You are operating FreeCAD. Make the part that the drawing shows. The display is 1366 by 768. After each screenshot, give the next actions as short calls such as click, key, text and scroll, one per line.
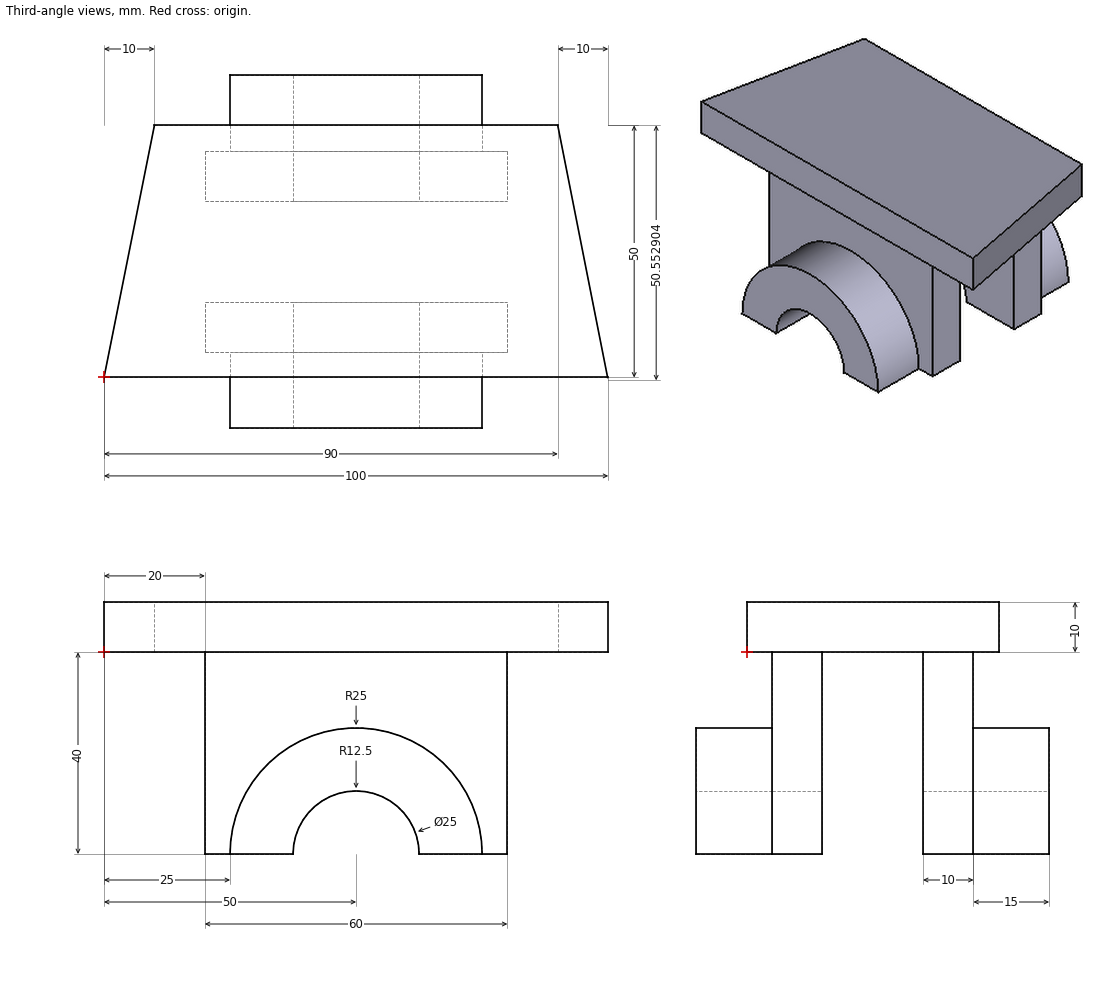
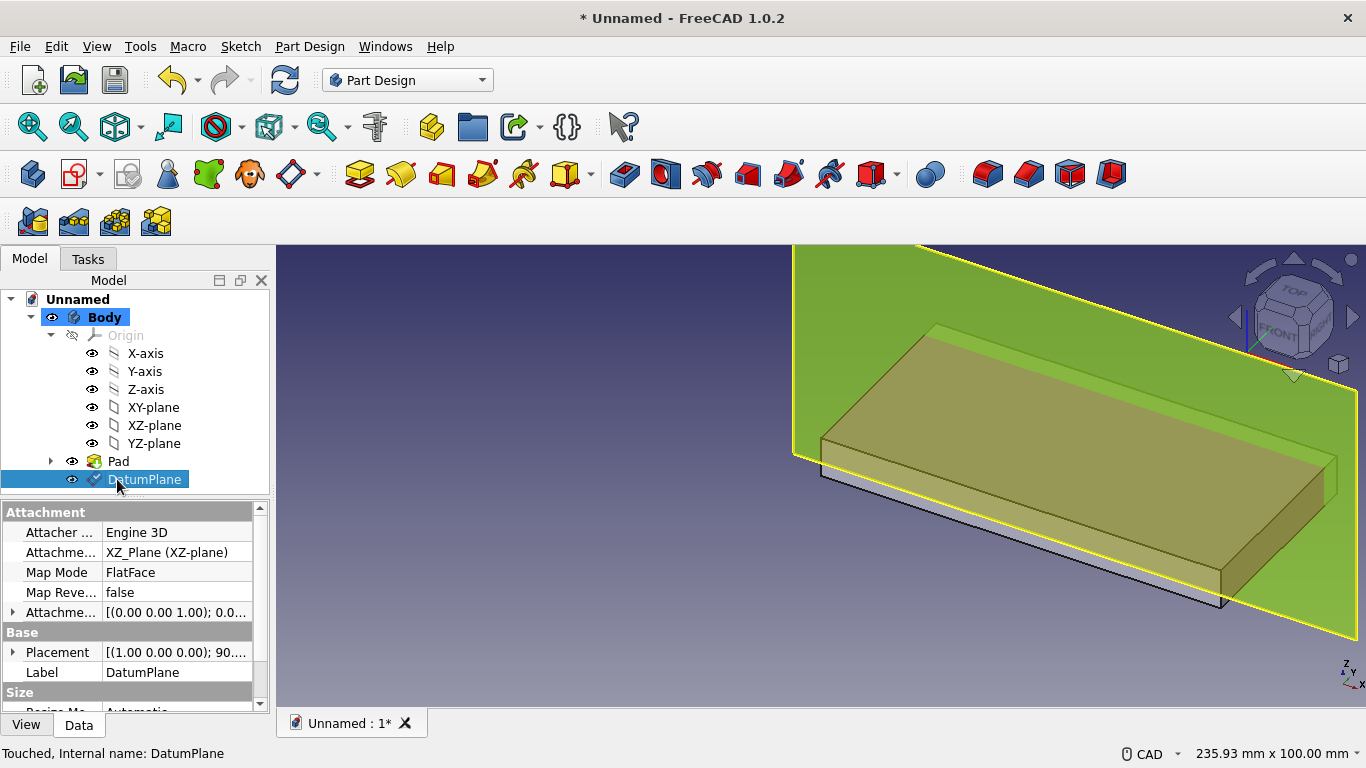
click(74, 174)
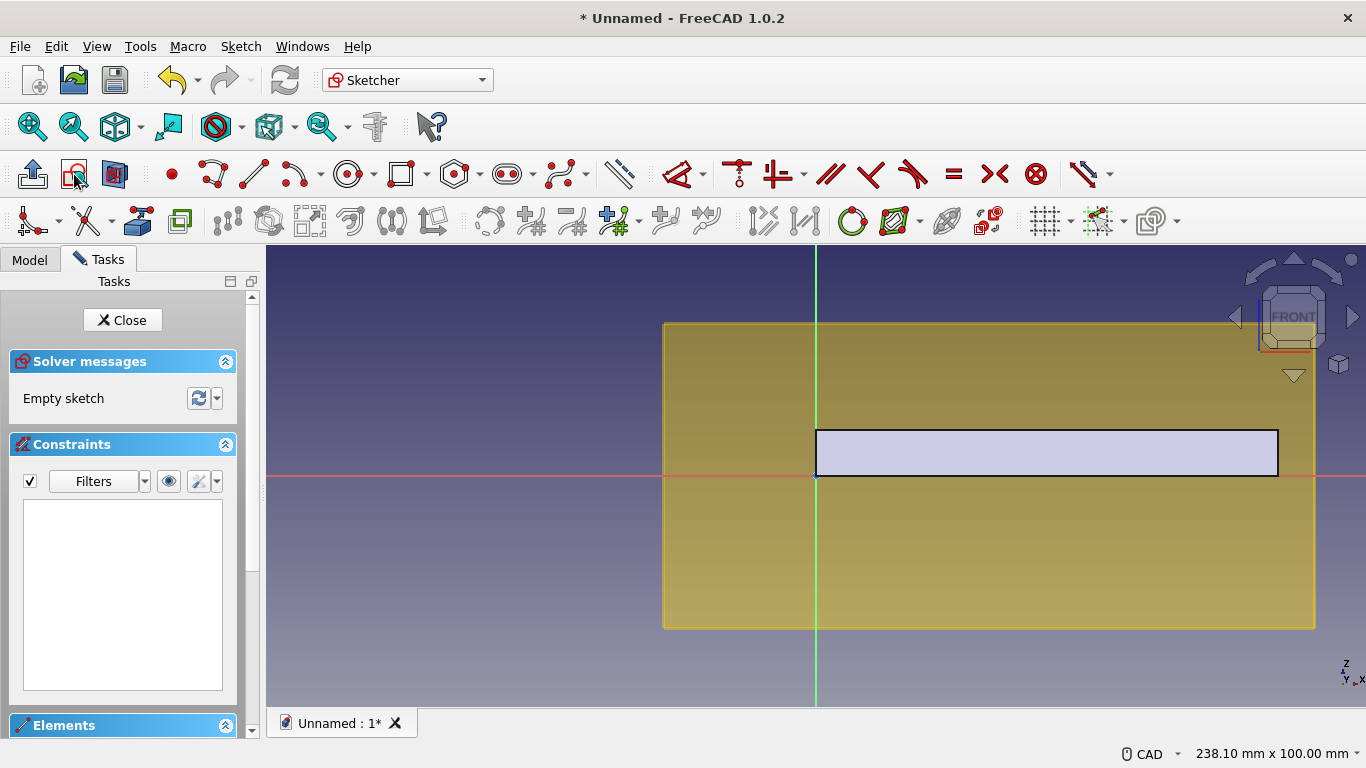
key(q)
key(s)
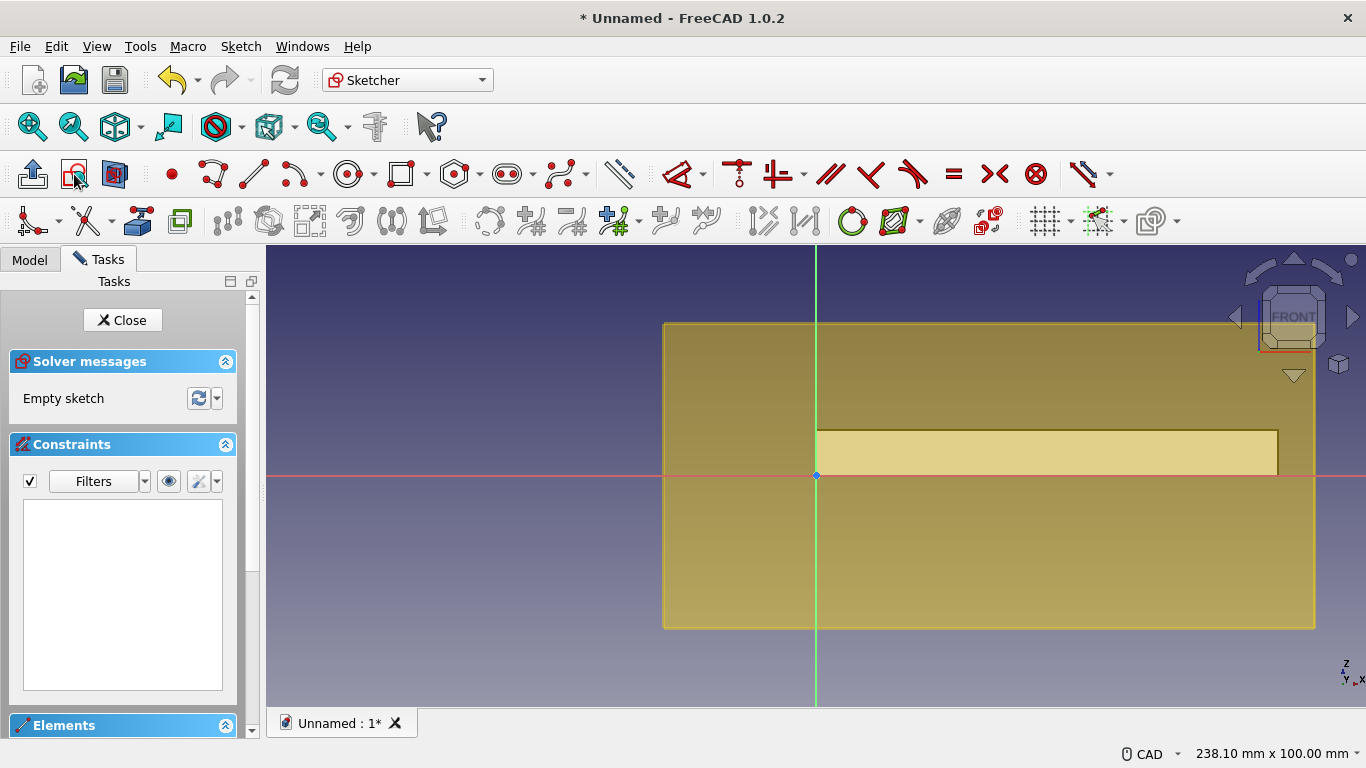
scroll(294, 273, down, 1)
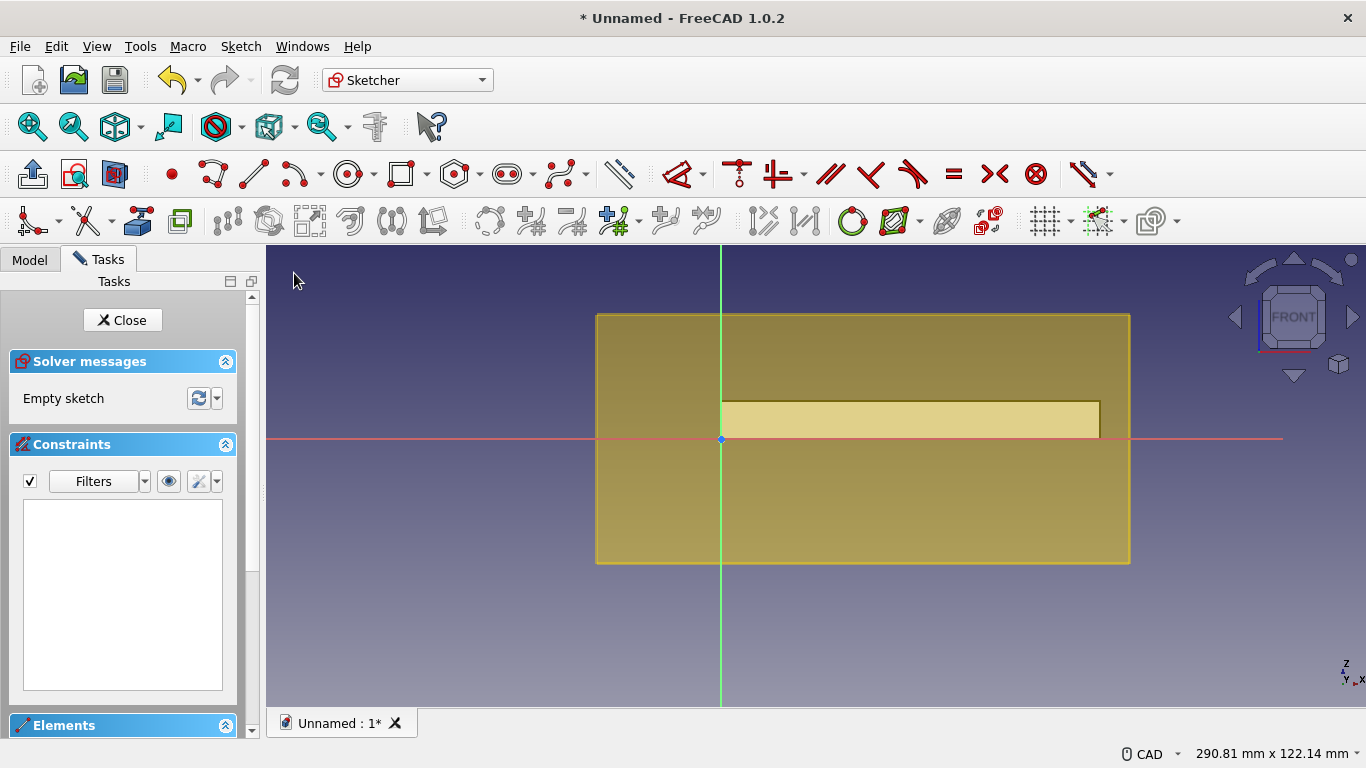
scroll(1025, 562, up, 3)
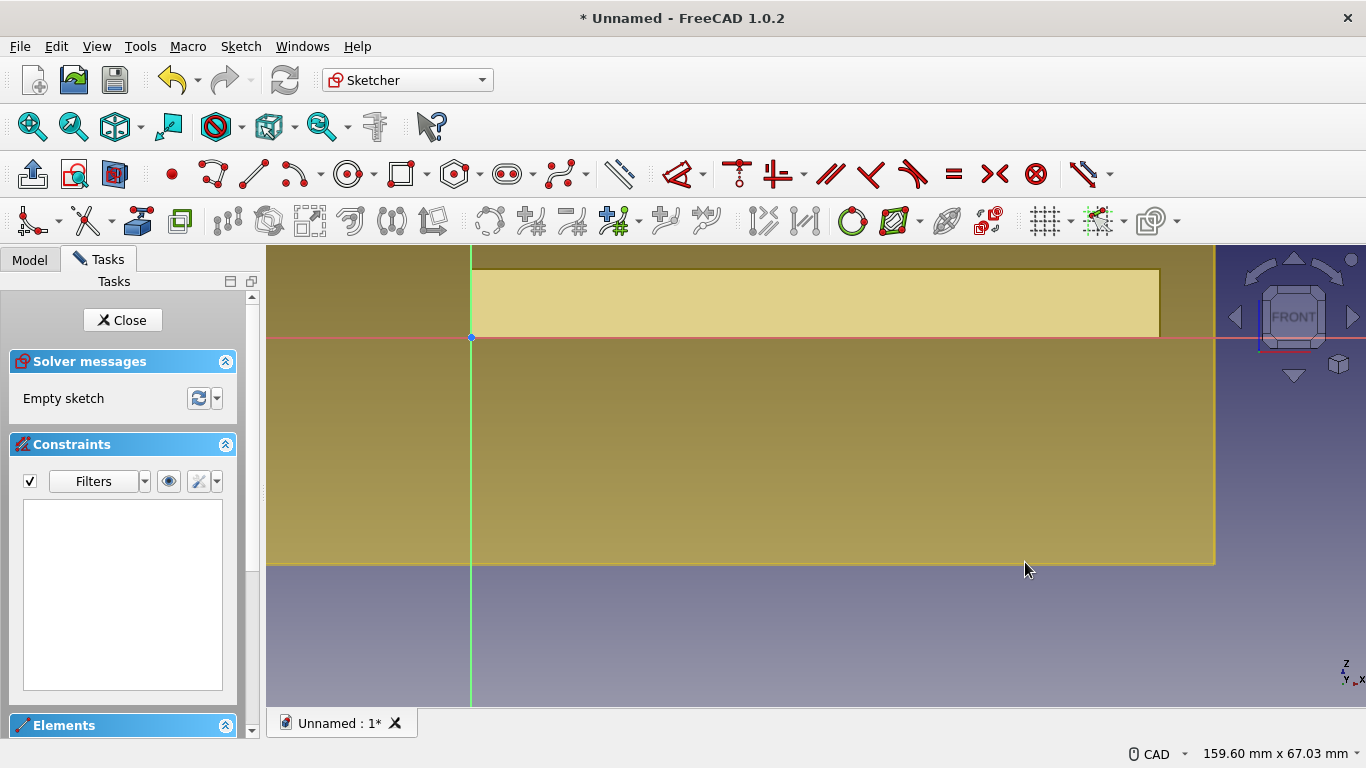
key(g)
key(r)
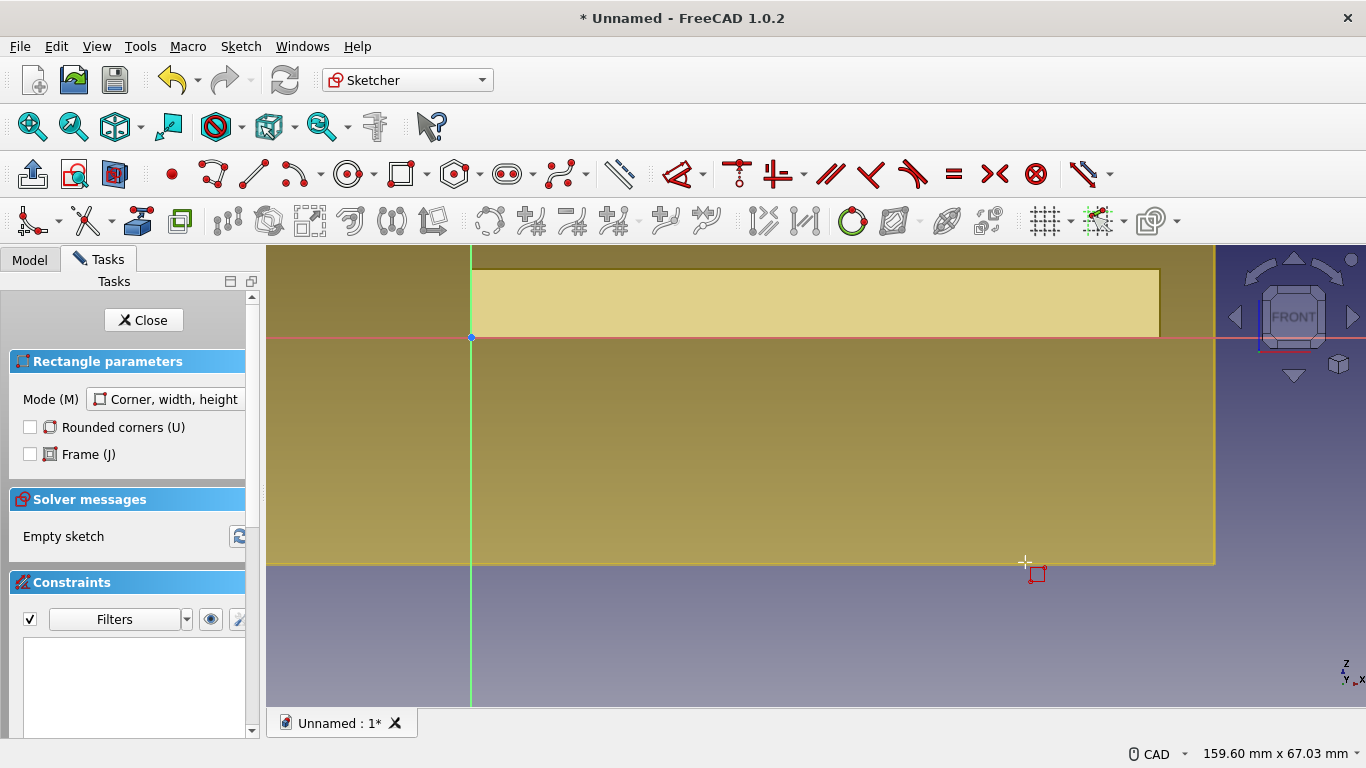
click(609, 338)
click(1023, 613)
key(Escape)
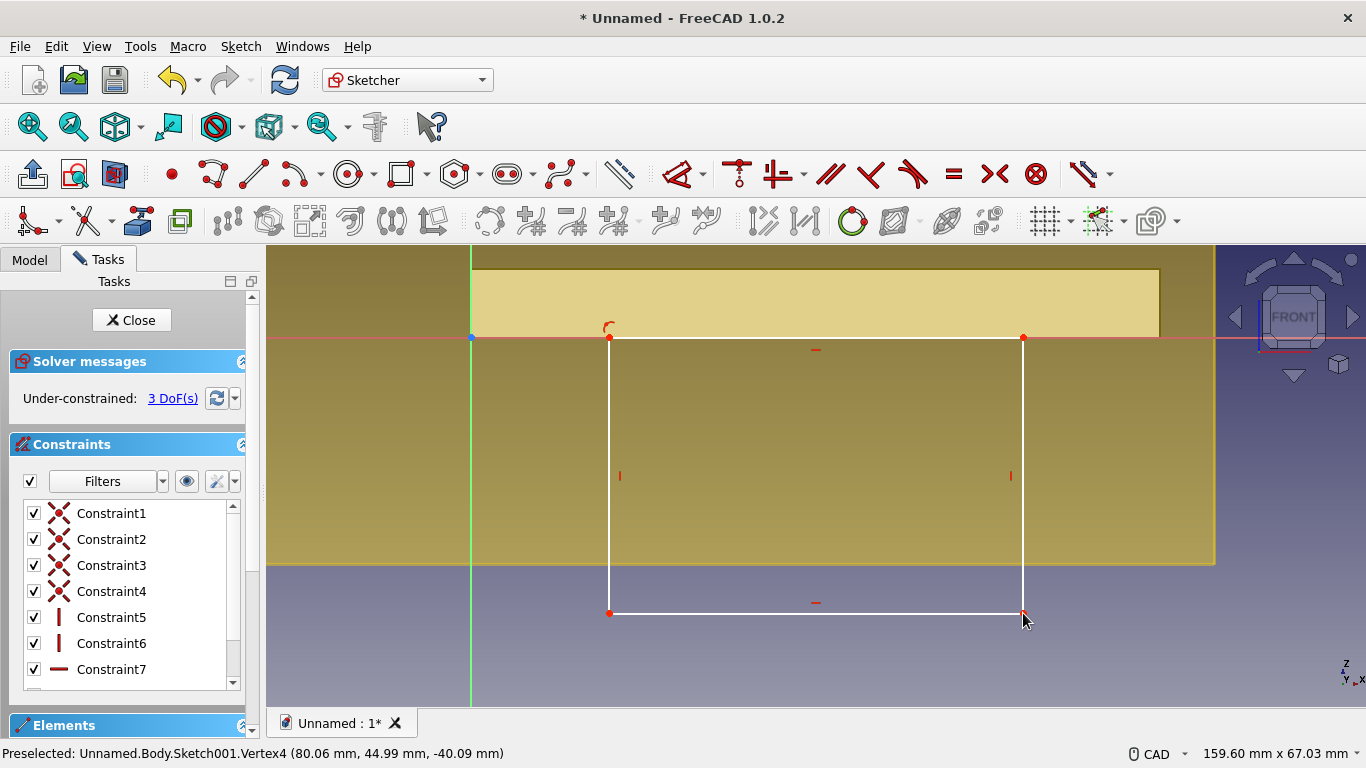
key(d)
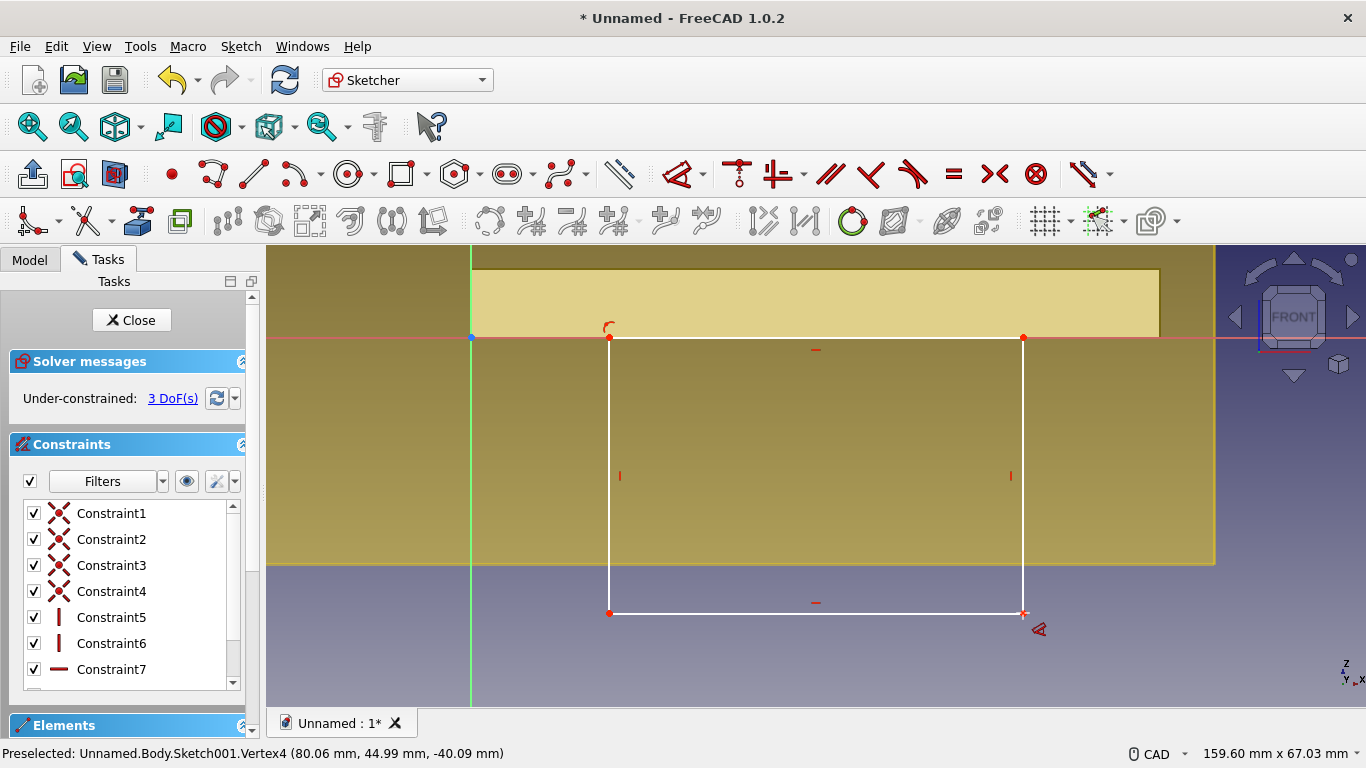
click(609, 421)
click(575, 476)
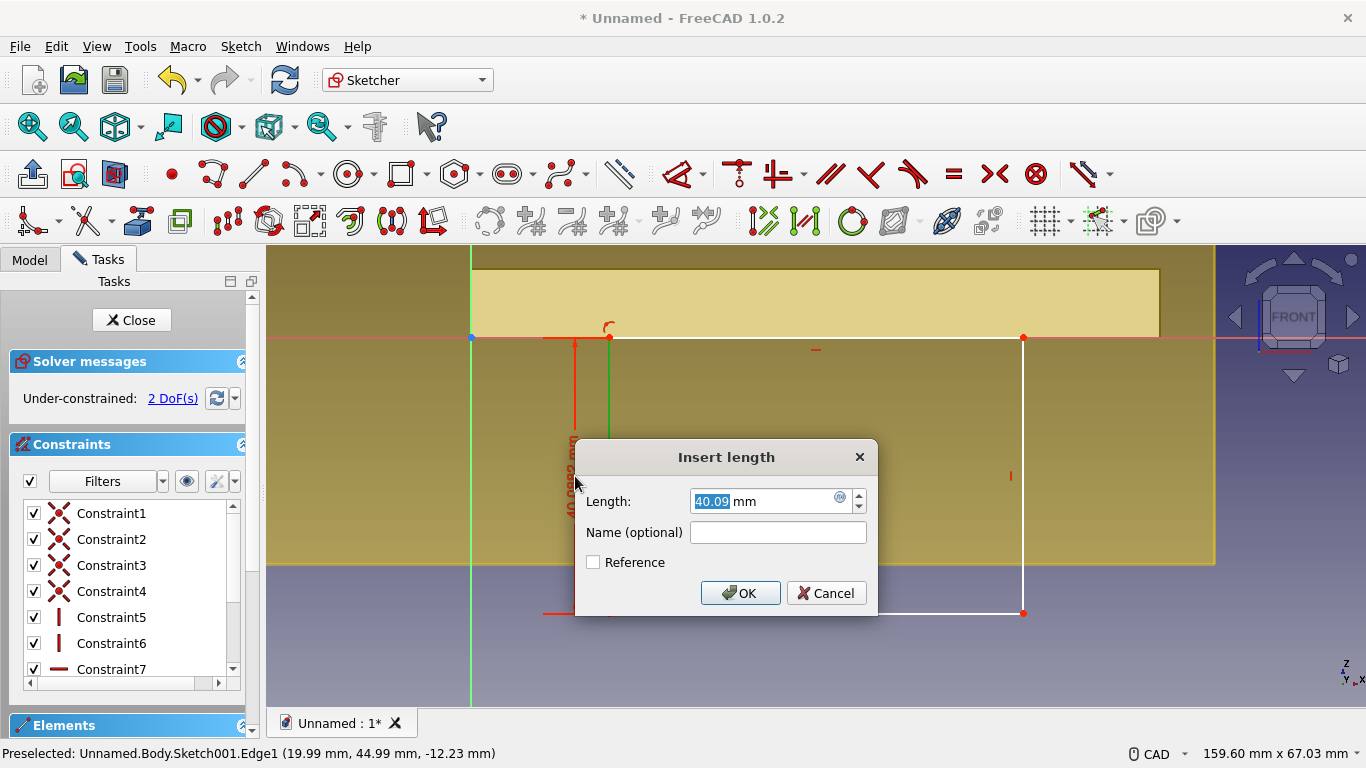
text(40)
key(Return)